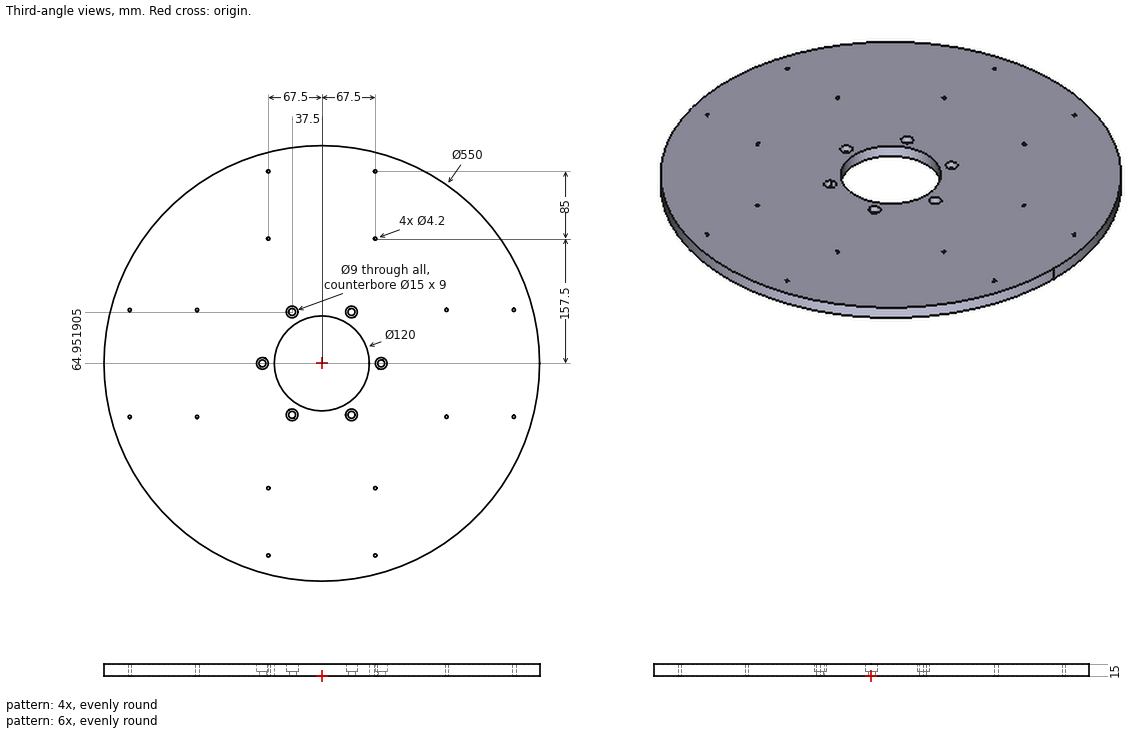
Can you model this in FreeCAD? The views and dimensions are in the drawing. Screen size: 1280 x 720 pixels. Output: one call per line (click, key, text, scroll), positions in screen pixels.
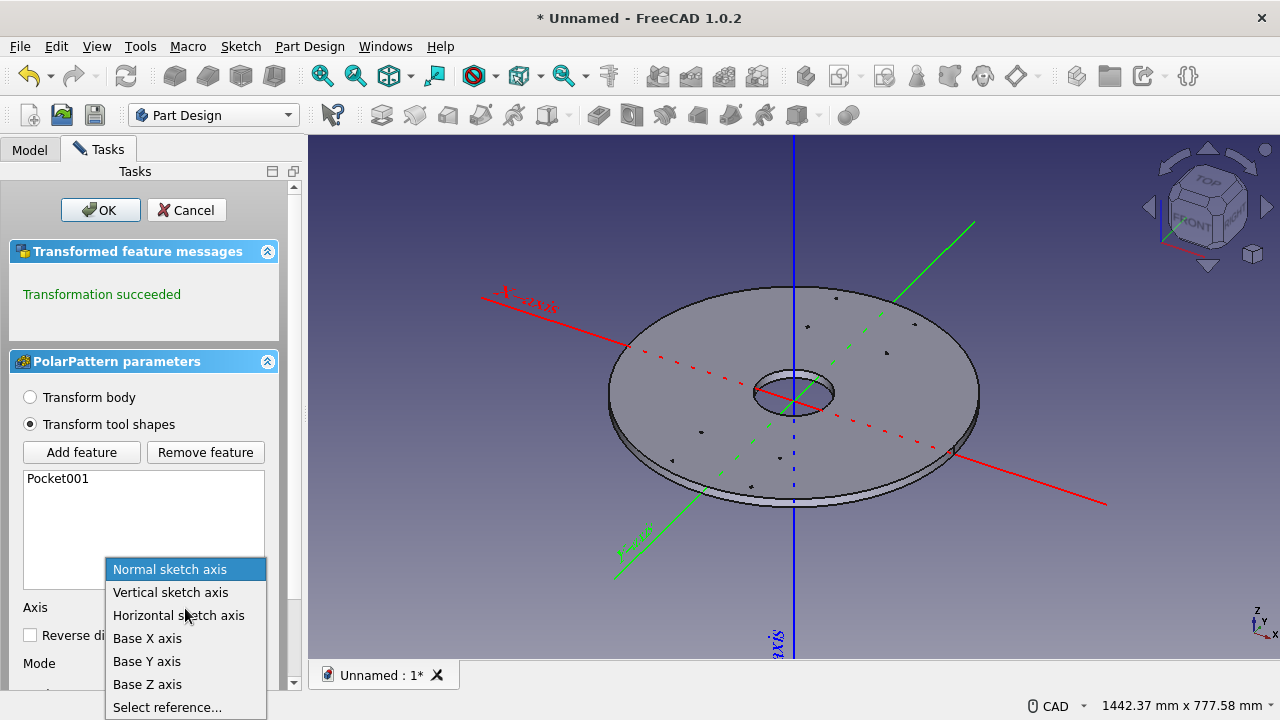
click(184, 684)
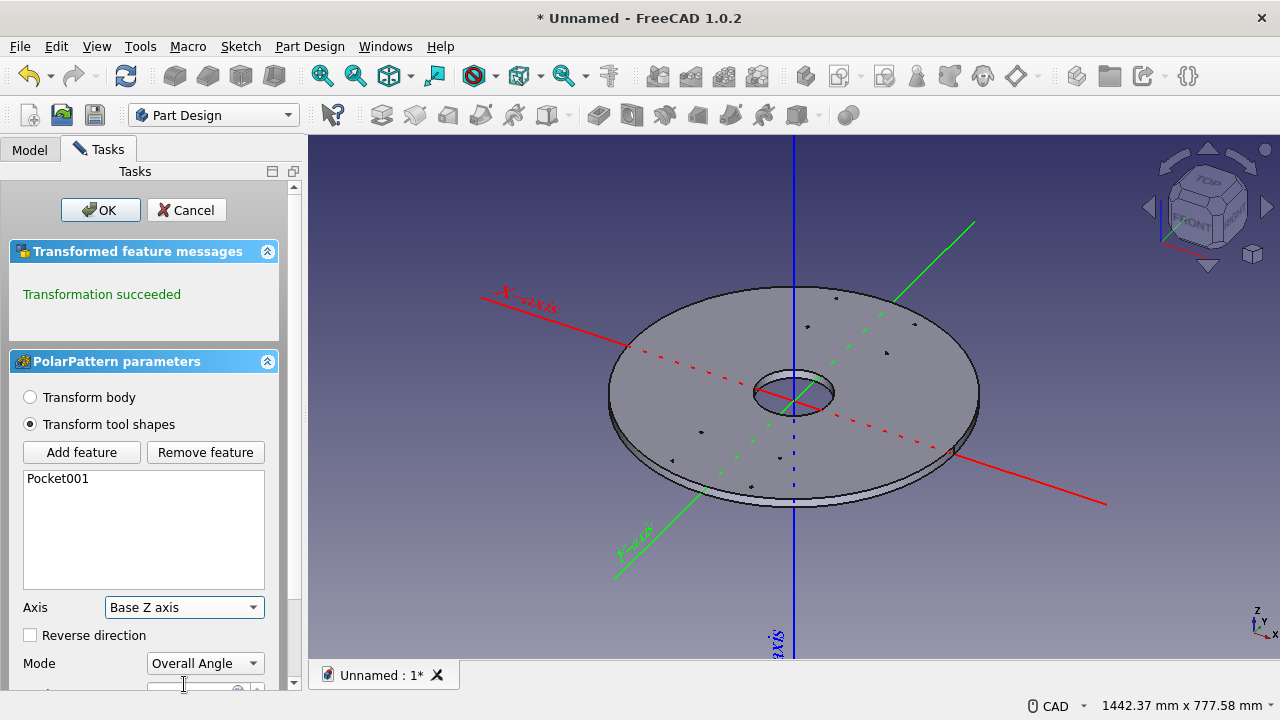
scroll(294, 436, down, 2)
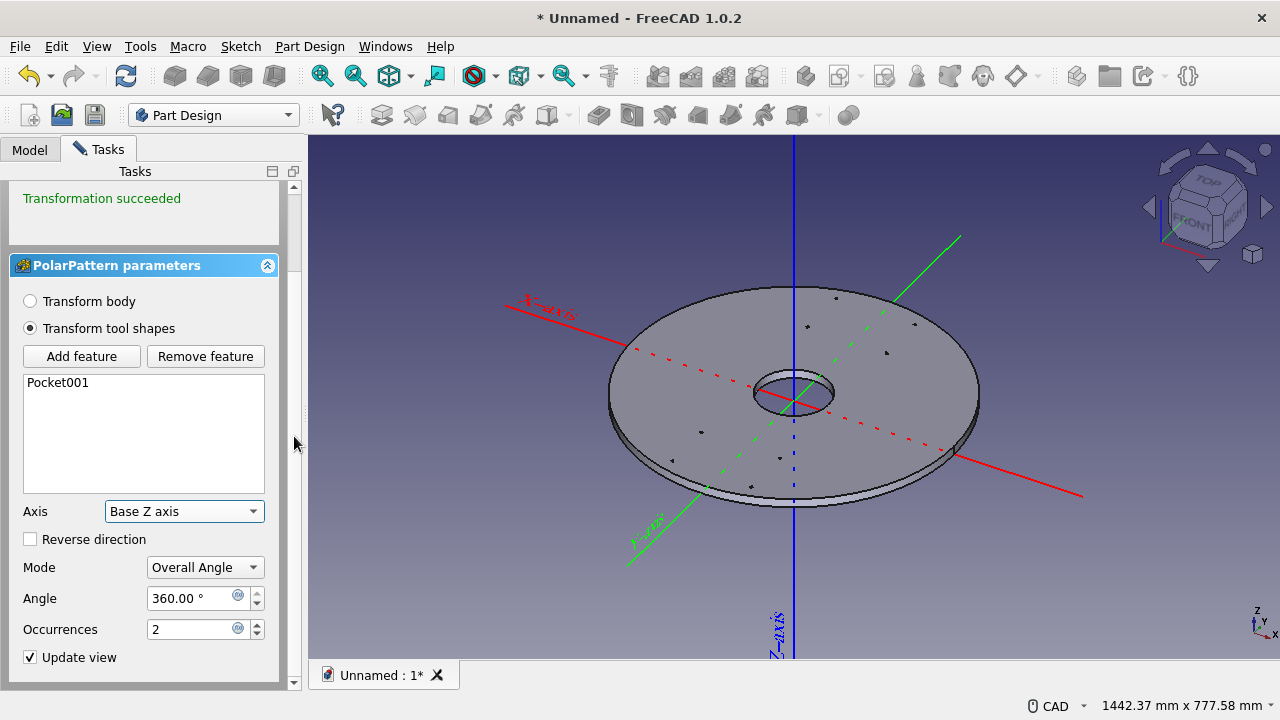
triple_click(199, 630)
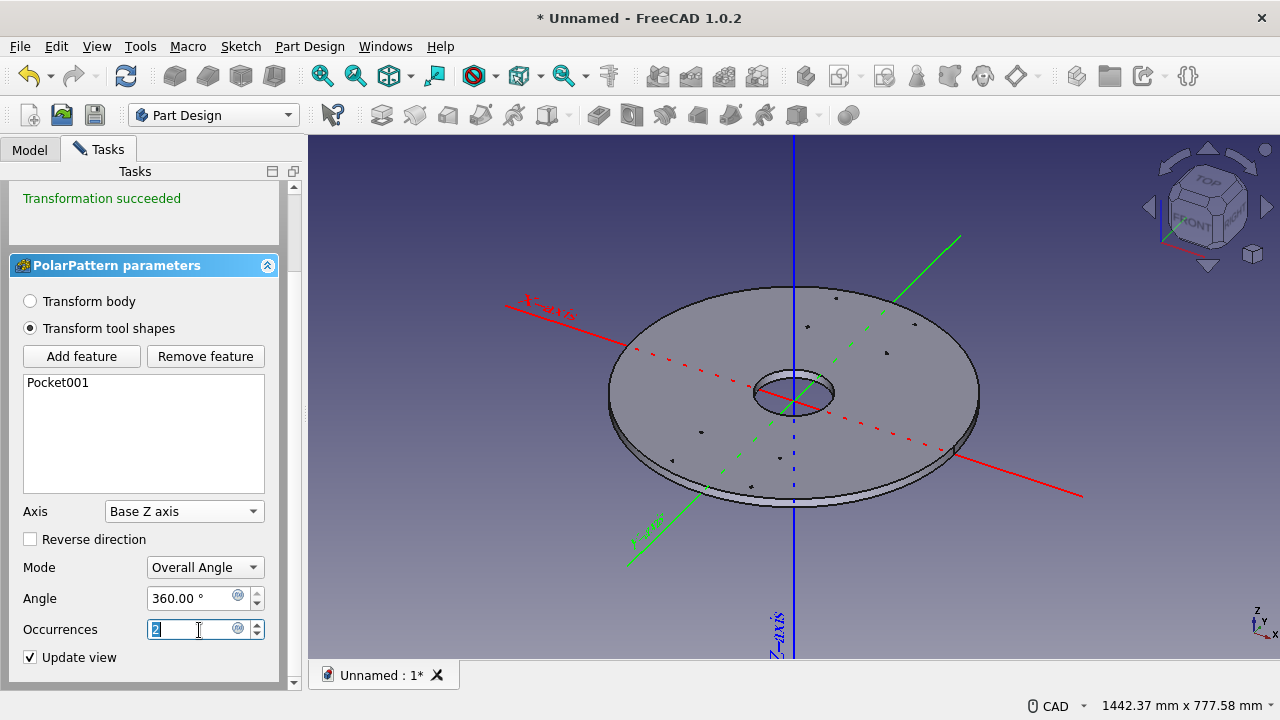
text(4)
key(Tab)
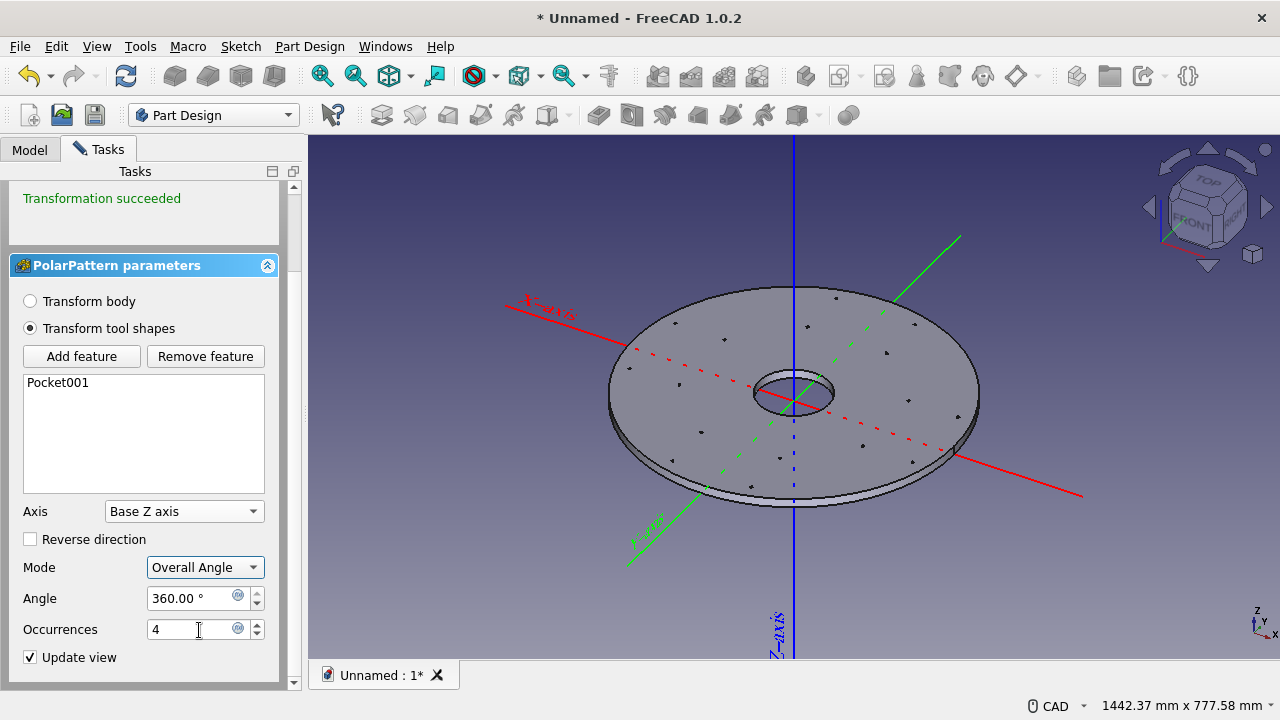
scroll(294, 436, up, 3)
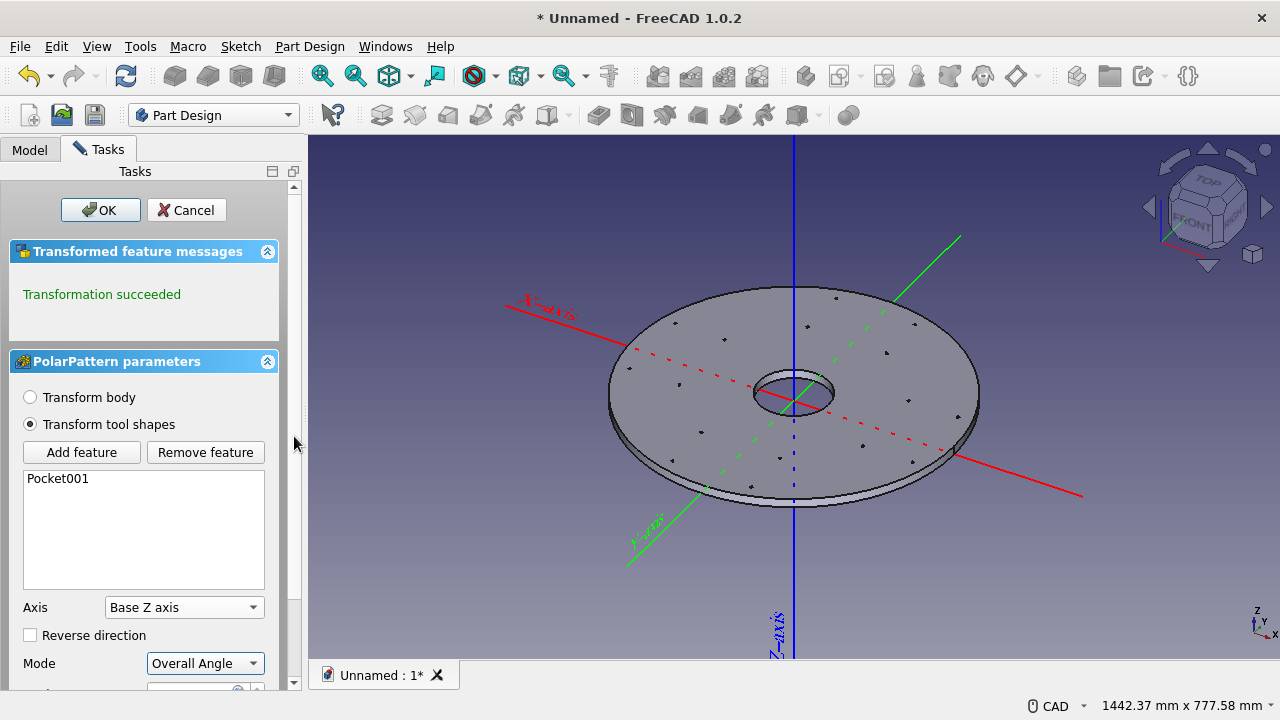
click(101, 210)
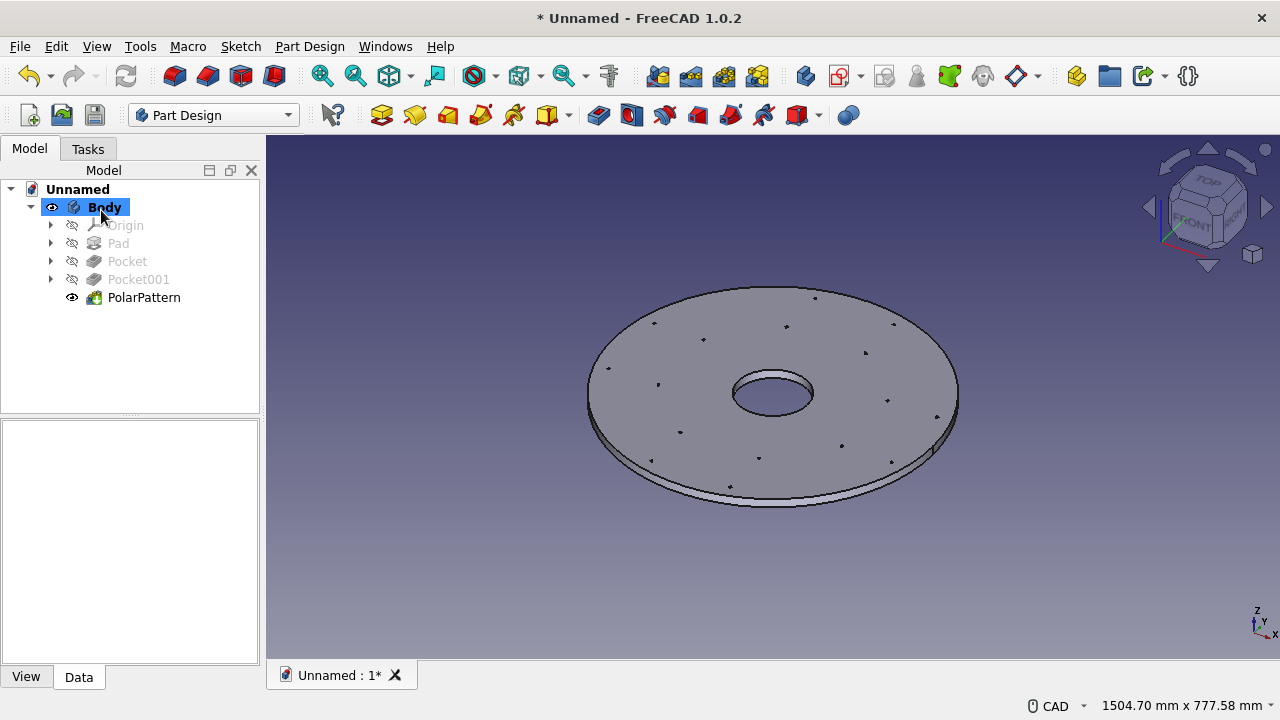
click(720, 444)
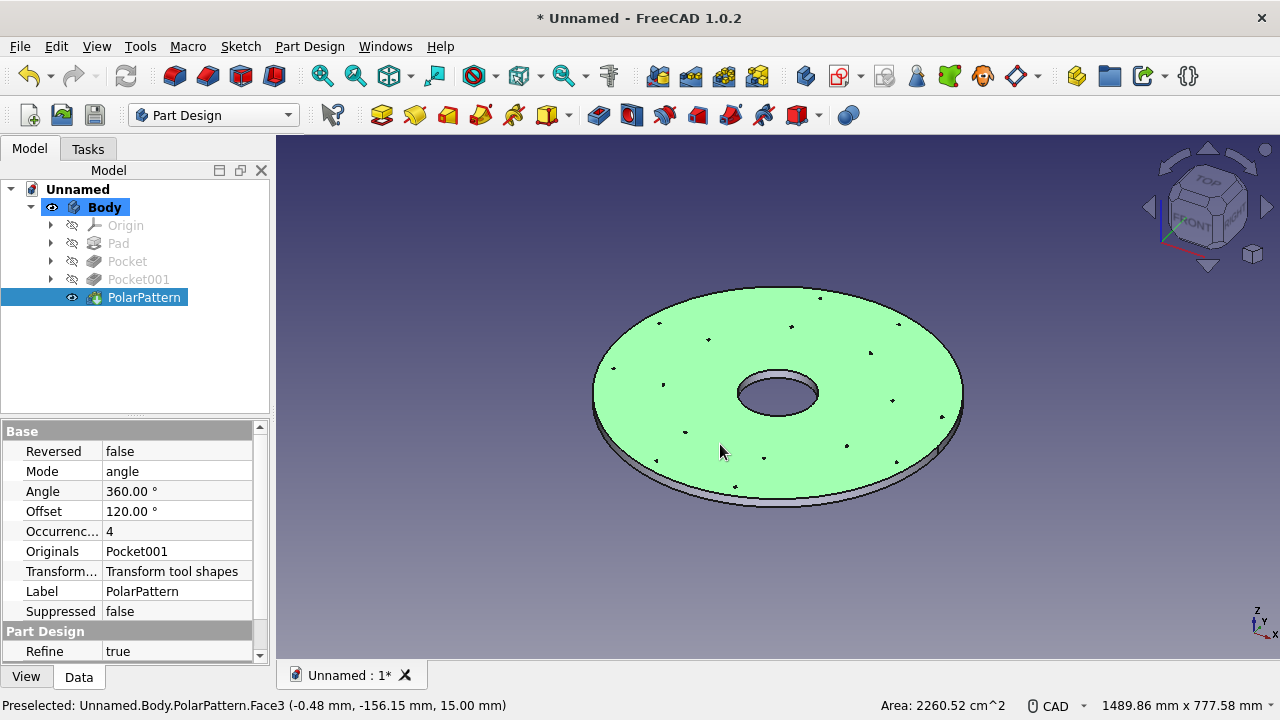
click(838, 76)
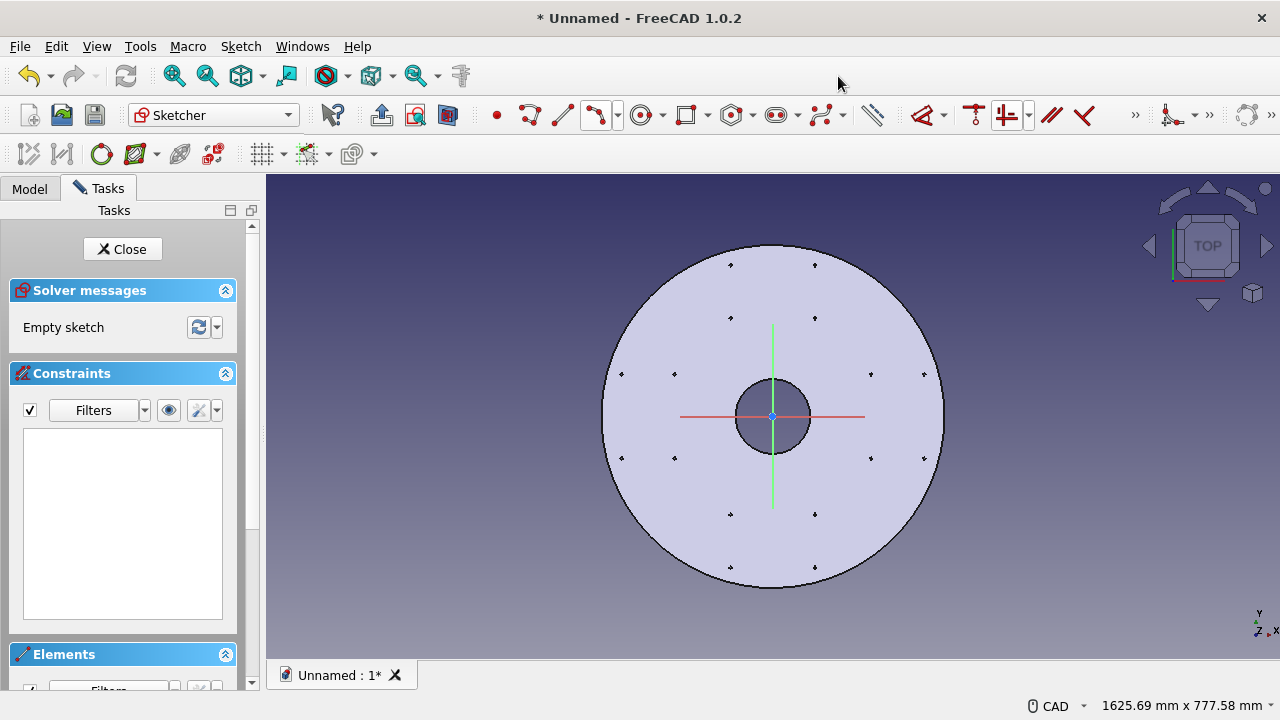
scroll(752, 374, up, 15)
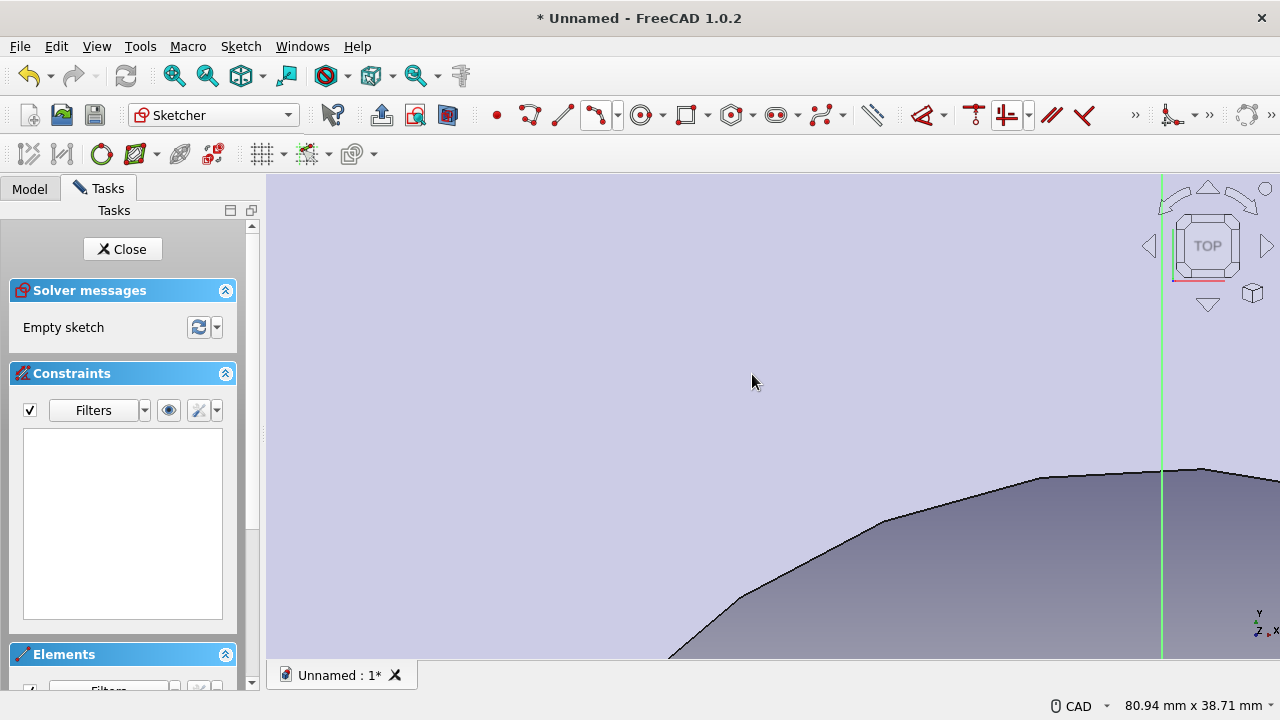
scroll(686, 400, up, 5)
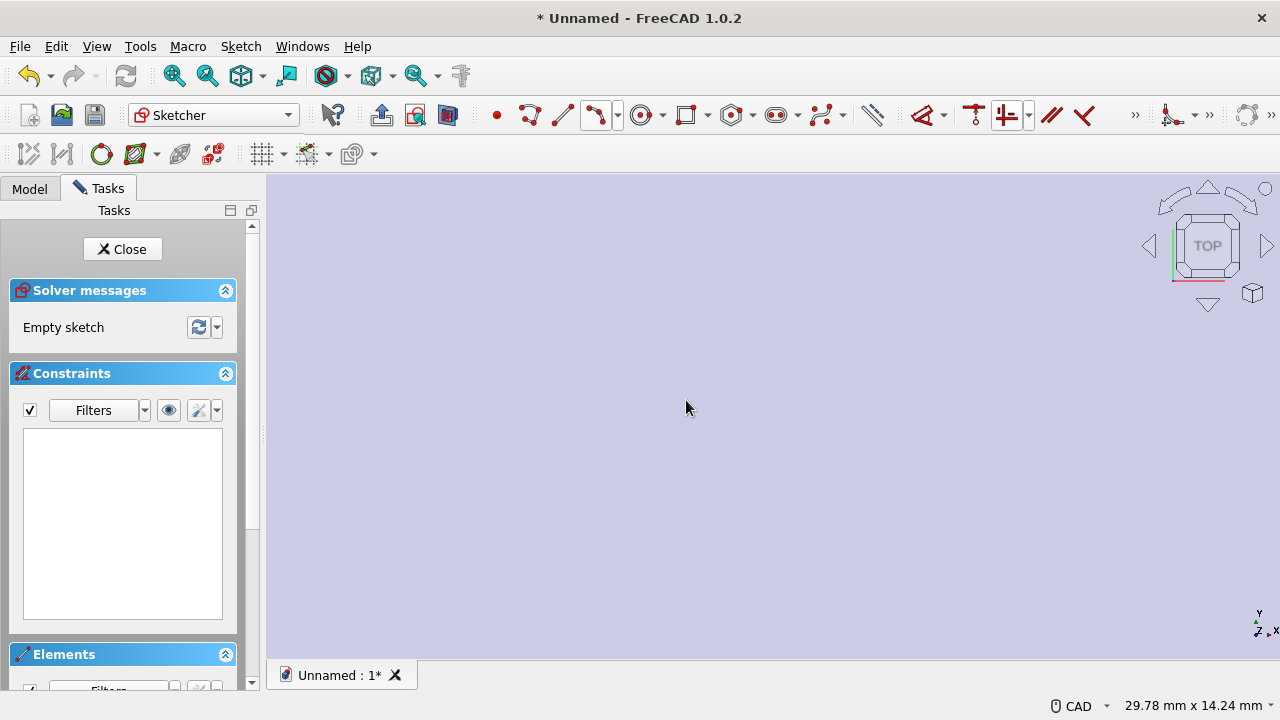
click(640, 116)